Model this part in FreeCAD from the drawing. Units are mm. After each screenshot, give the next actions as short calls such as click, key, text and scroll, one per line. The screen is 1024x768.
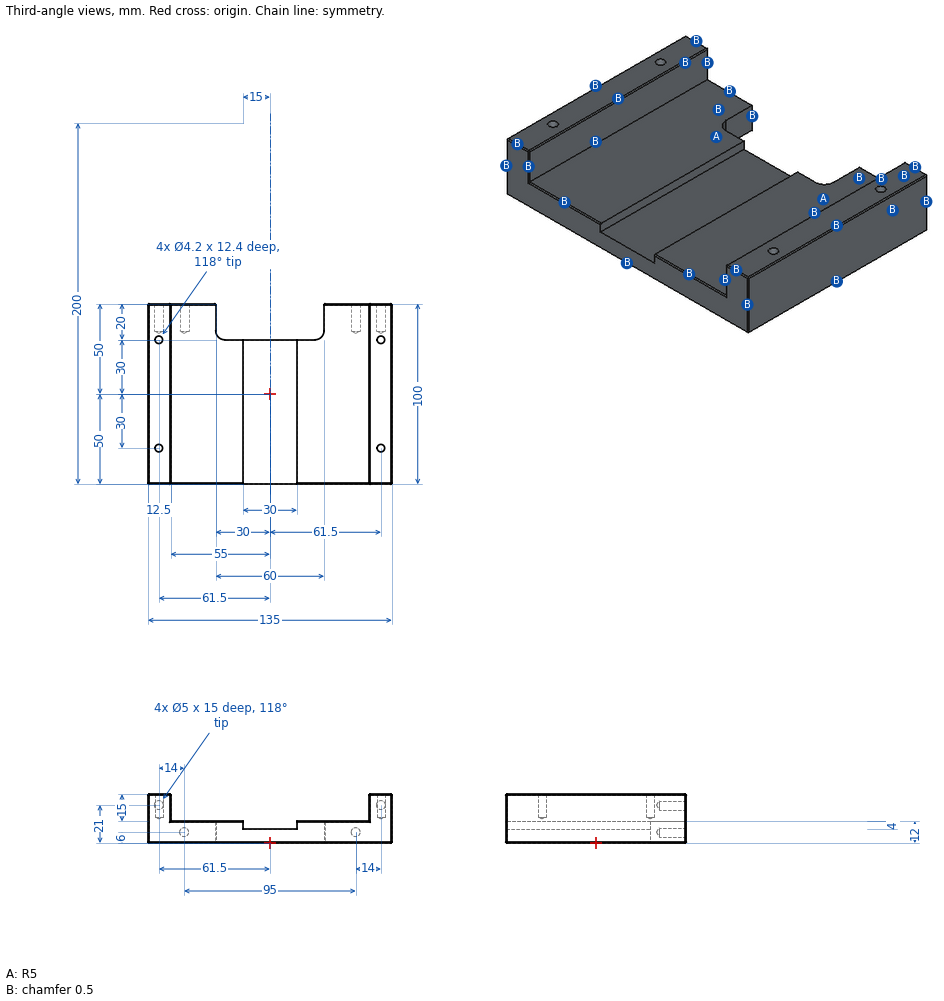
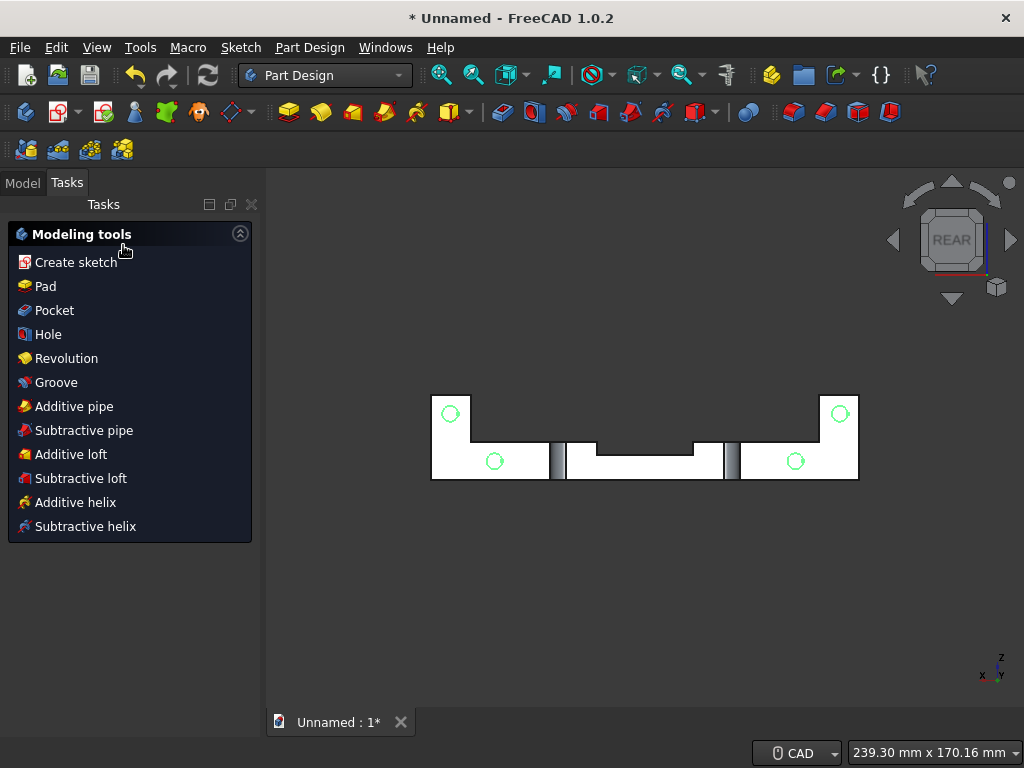
click(536, 112)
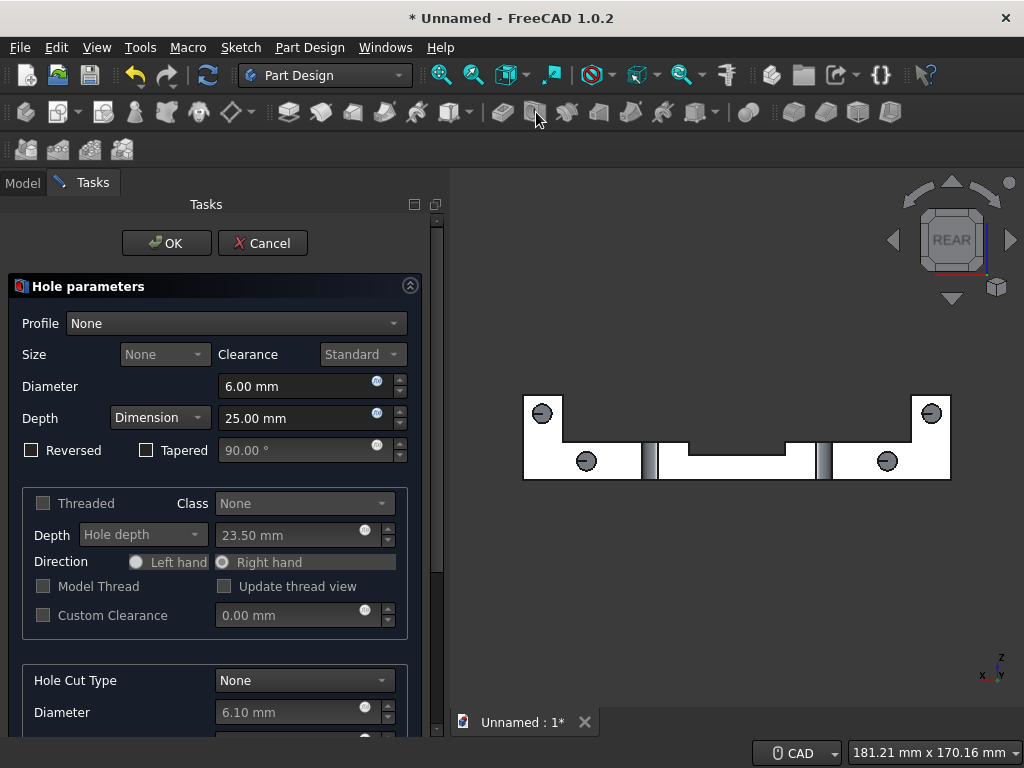
triple_click(305, 386)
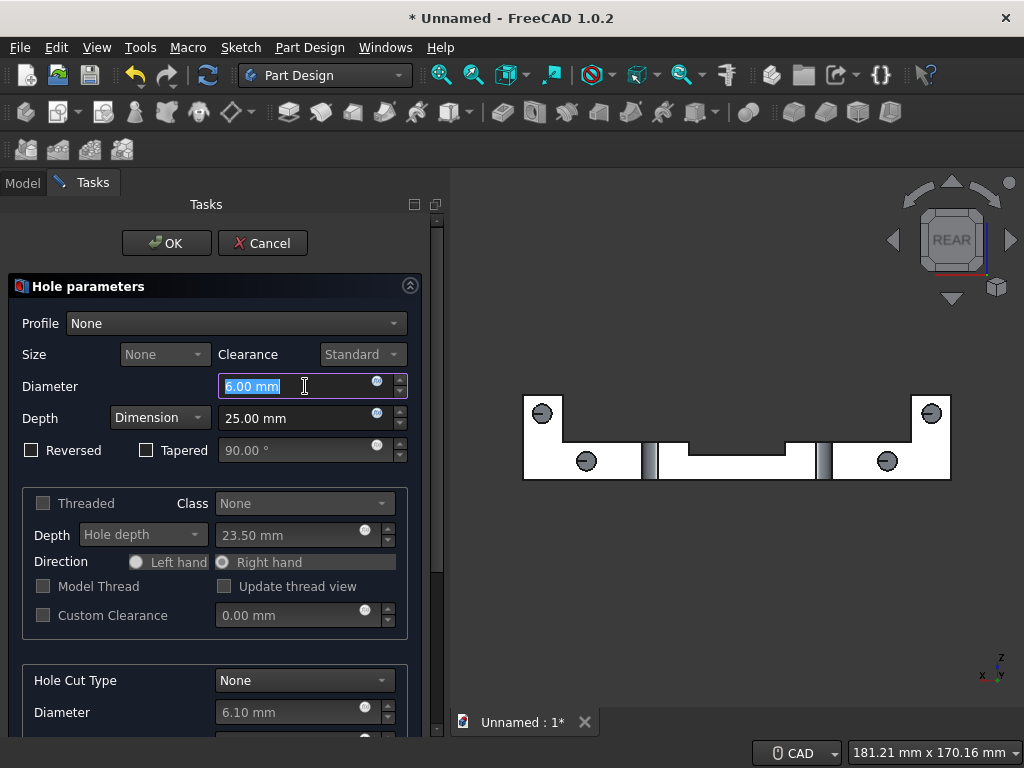
text(5)
key(Tab)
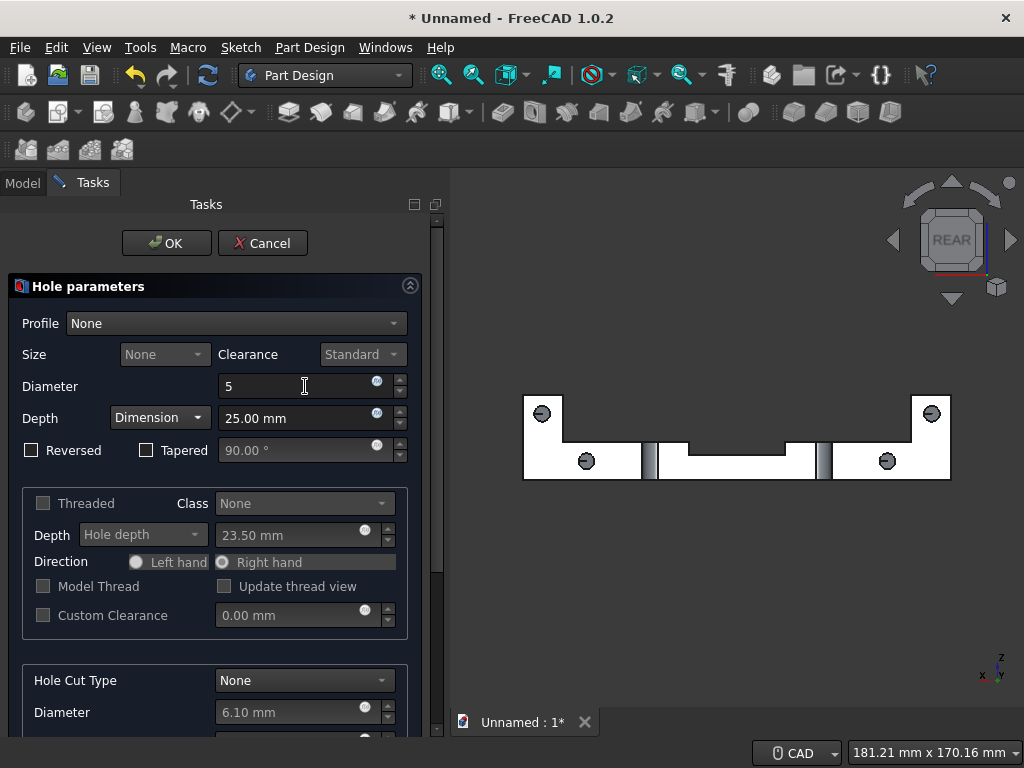
triple_click(305, 418)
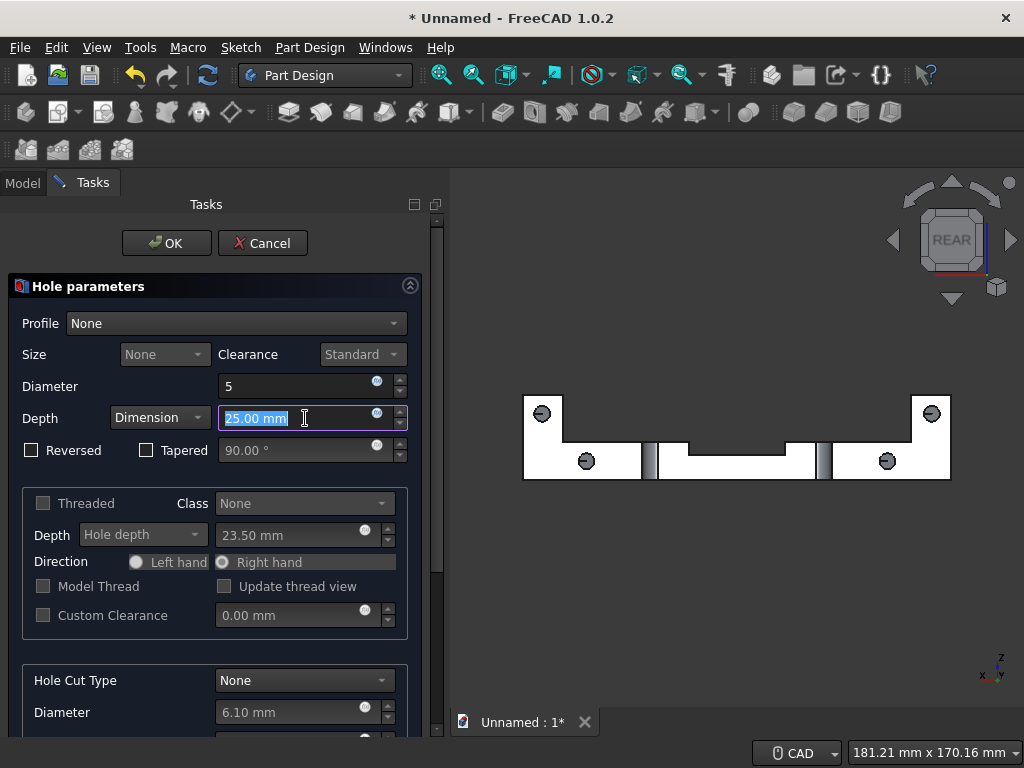
text(15)
key(Tab)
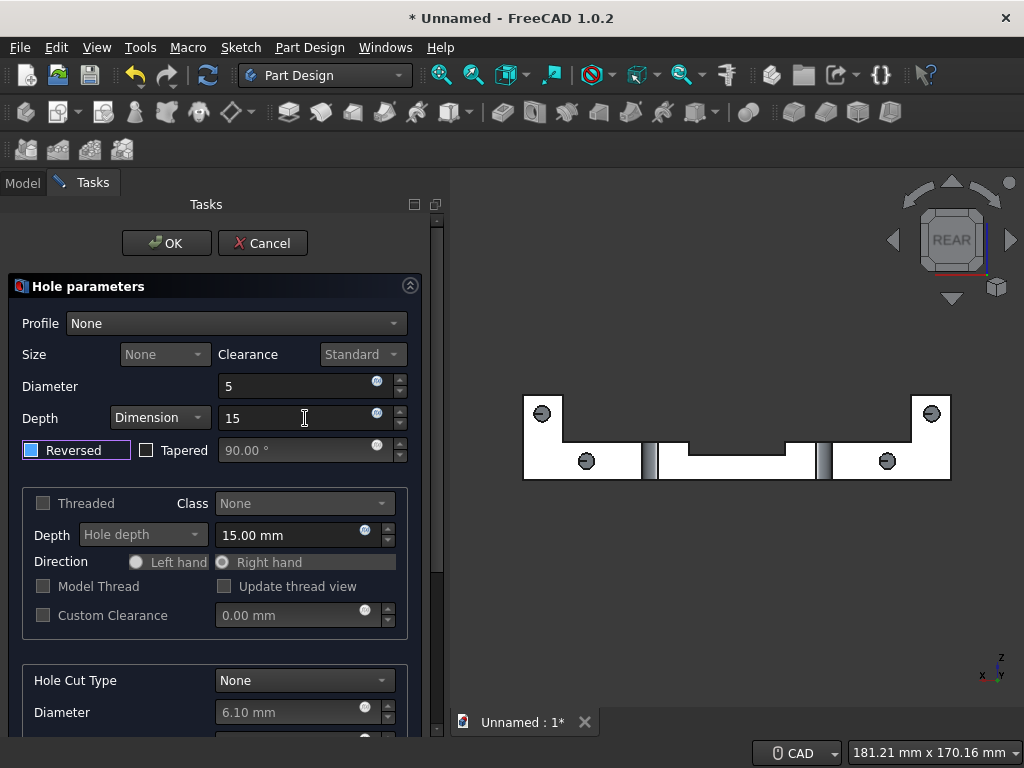
click(167, 243)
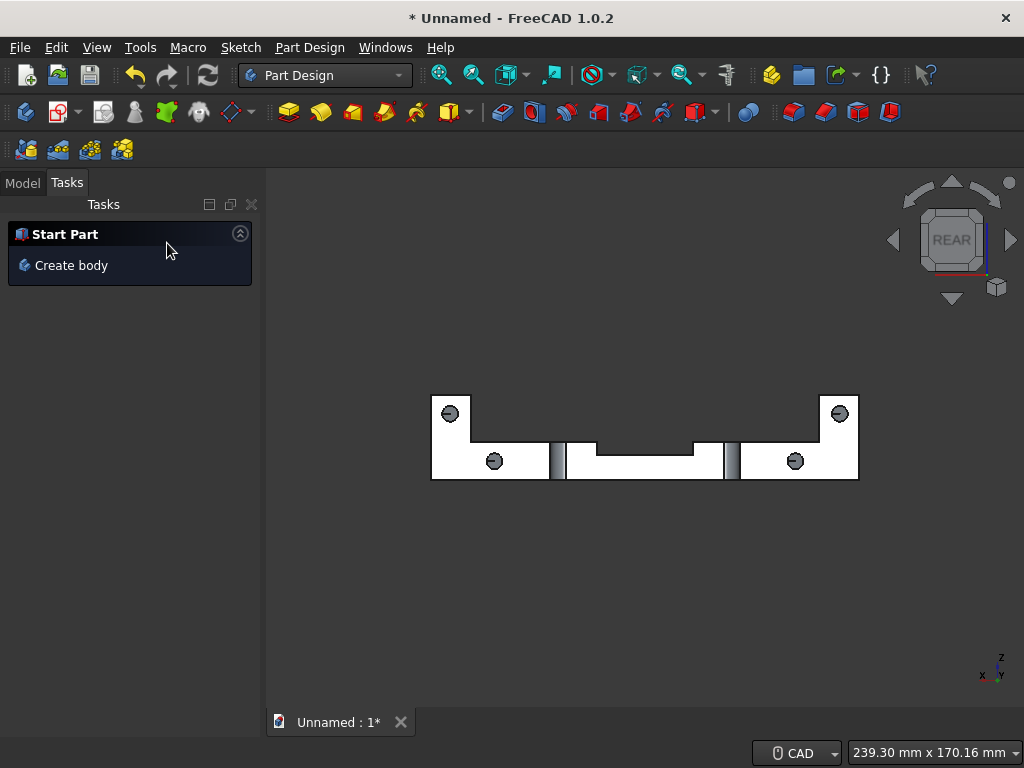
key(0)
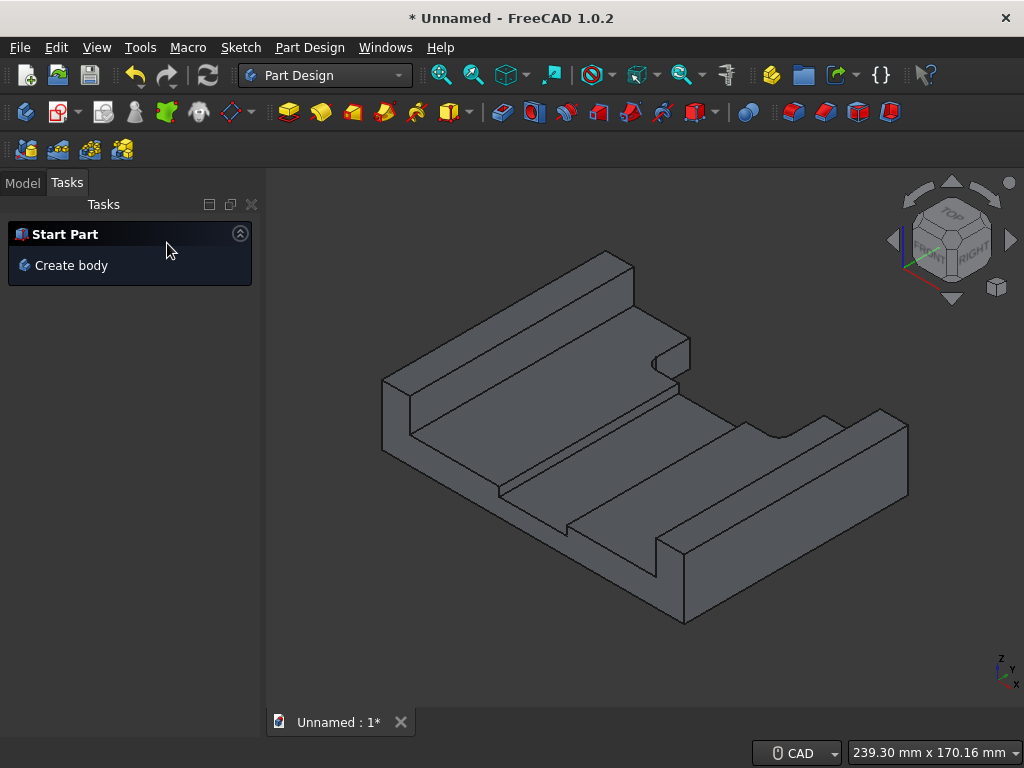
click(878, 425)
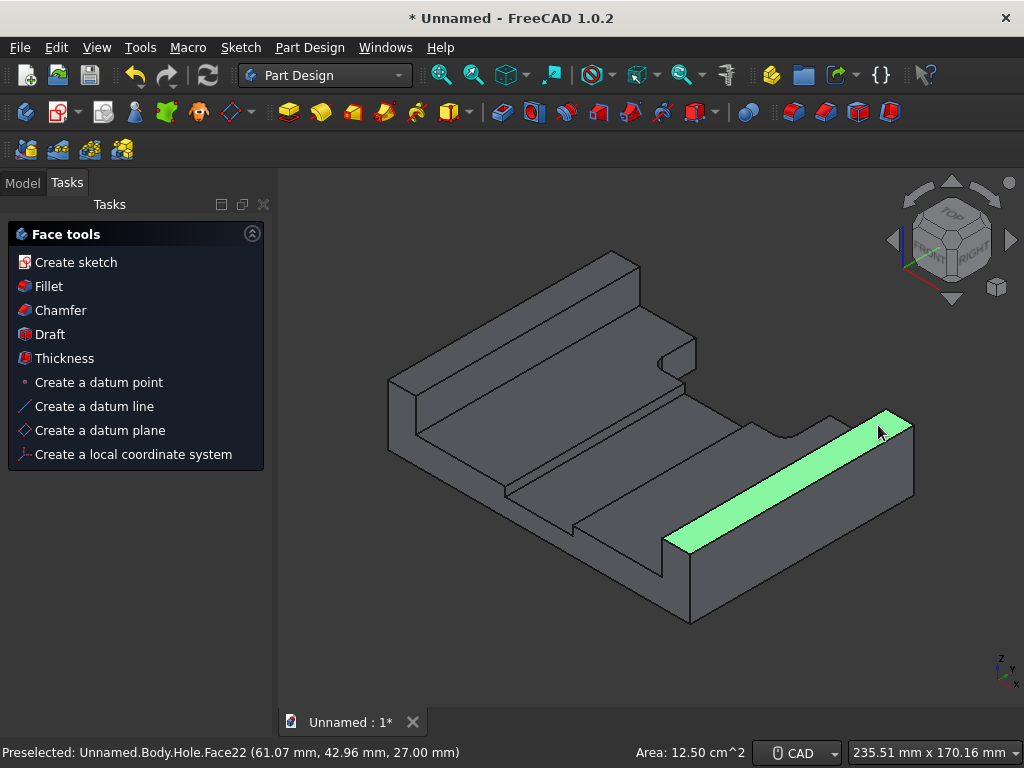
click(58, 112)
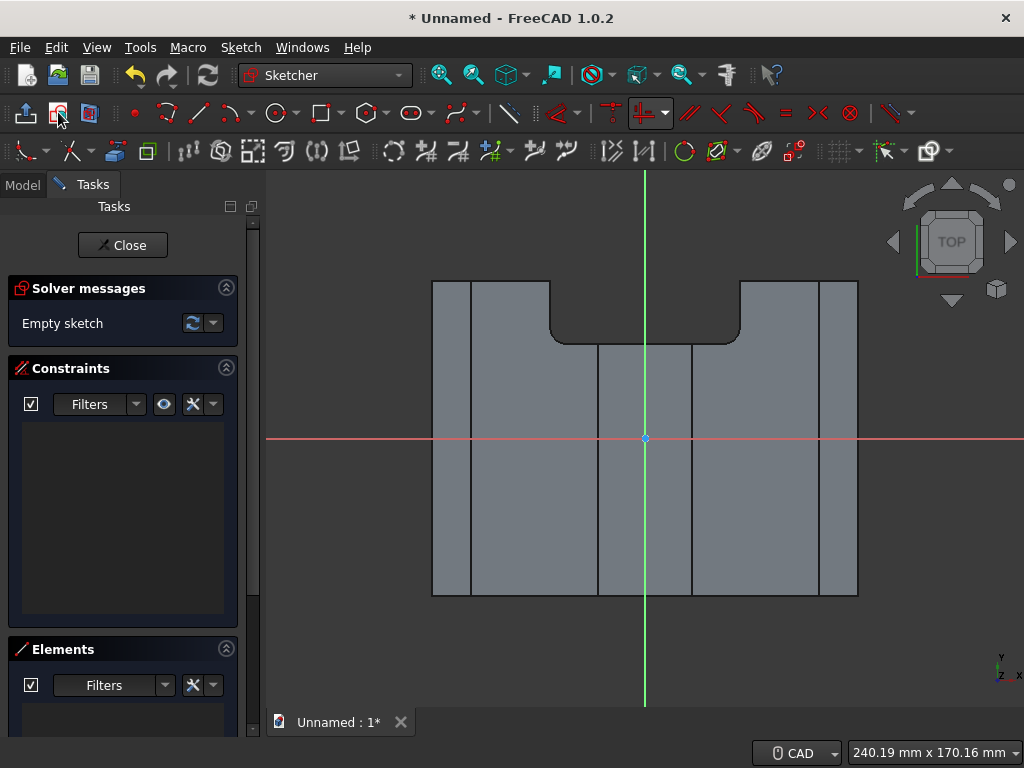
scroll(294, 439, down, 1)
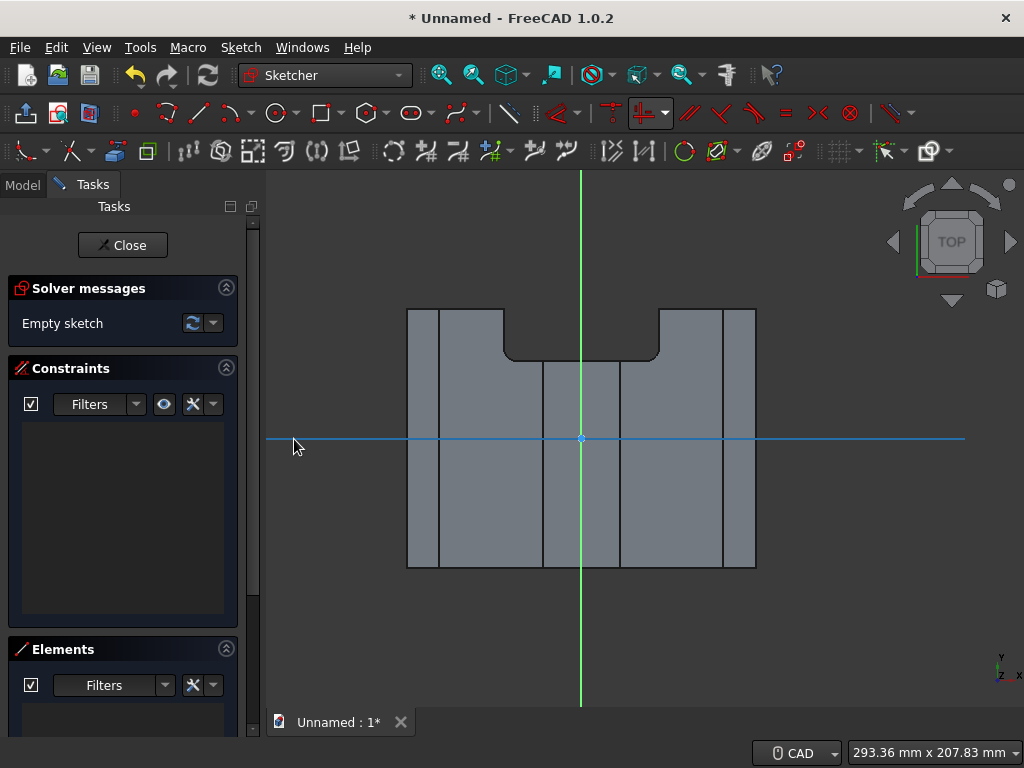
click(276, 114)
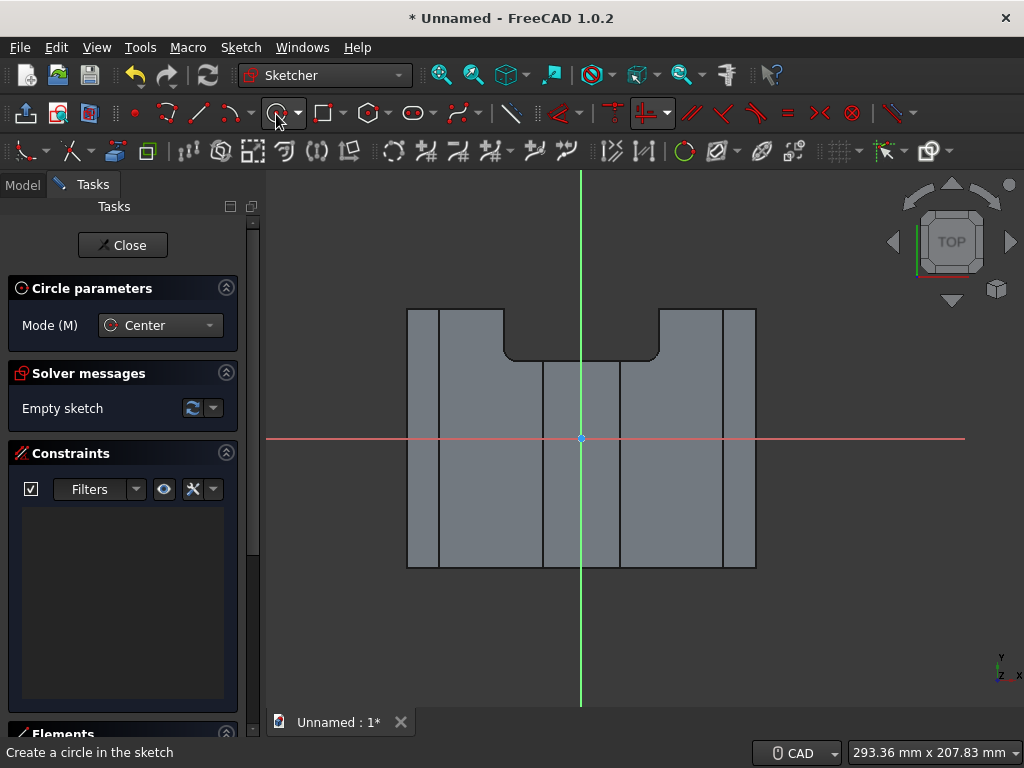
scroll(422, 361, up, 8)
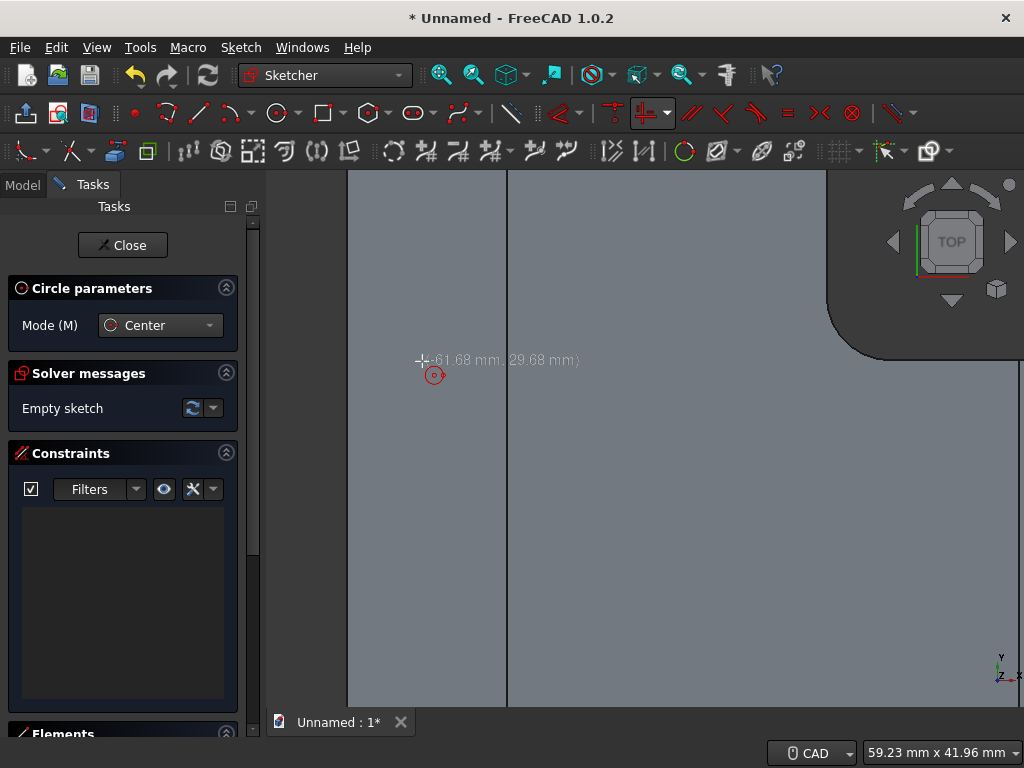
scroll(369, 338, down, 7)